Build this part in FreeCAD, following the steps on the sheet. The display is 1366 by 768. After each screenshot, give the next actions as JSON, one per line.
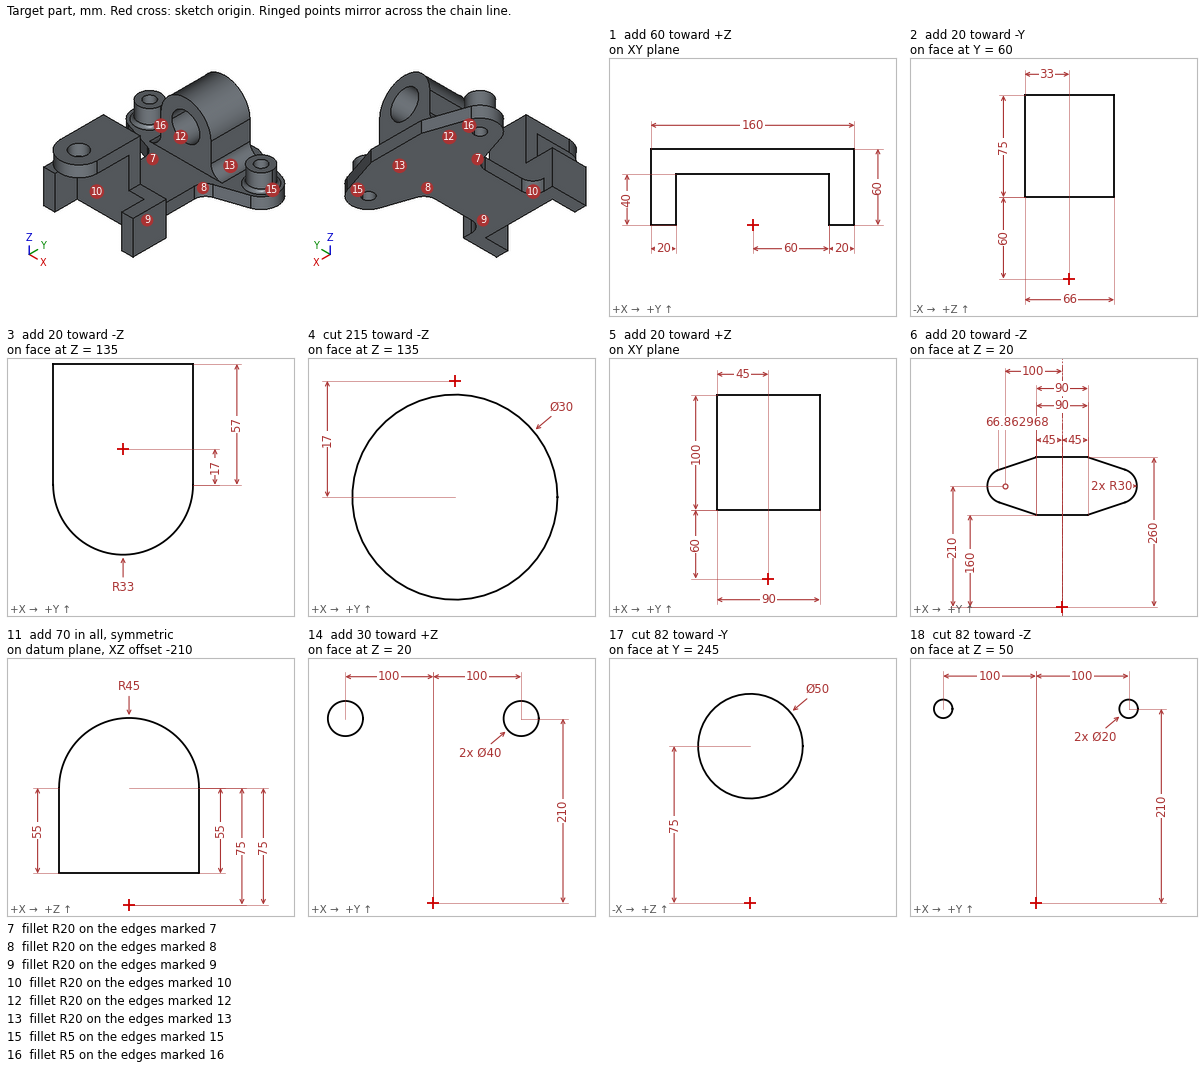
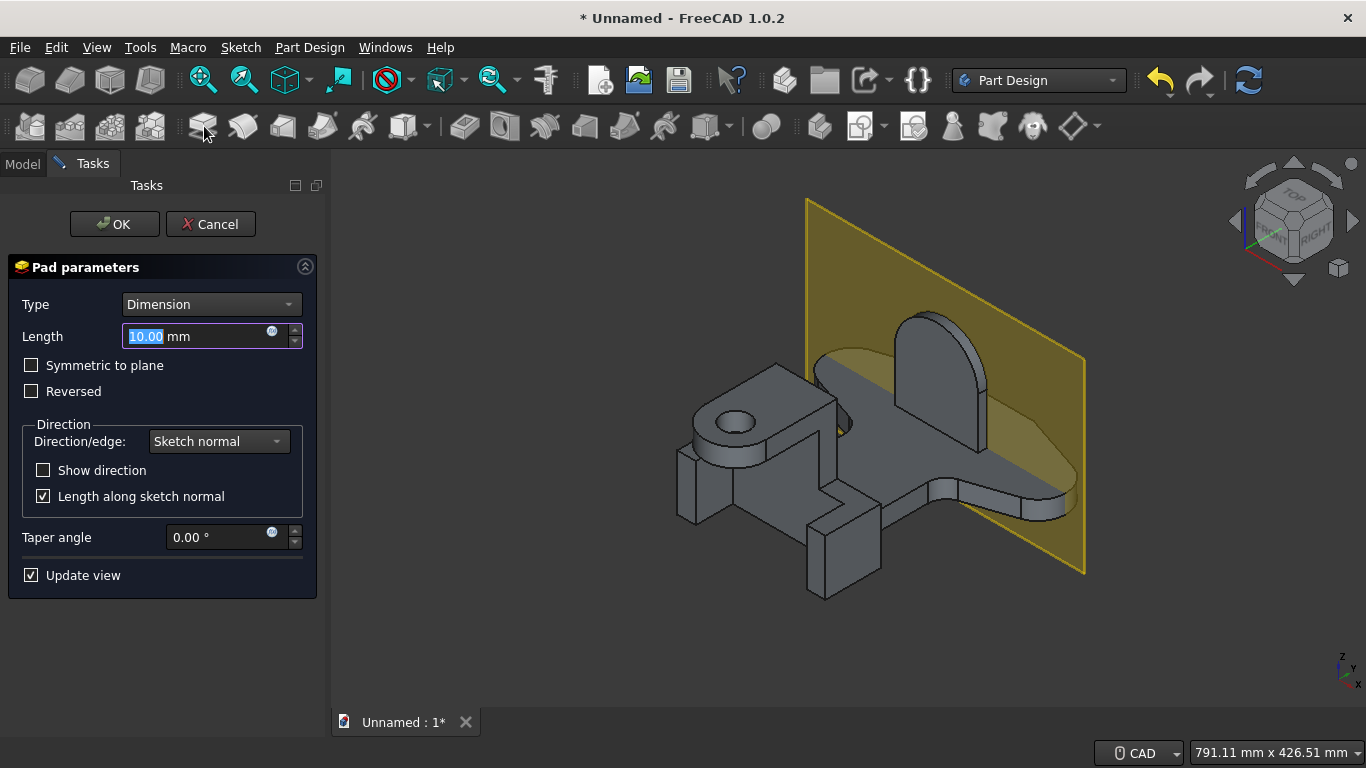
{"action": "type", "text": "70"}
{"action": "key", "text": "Tab"}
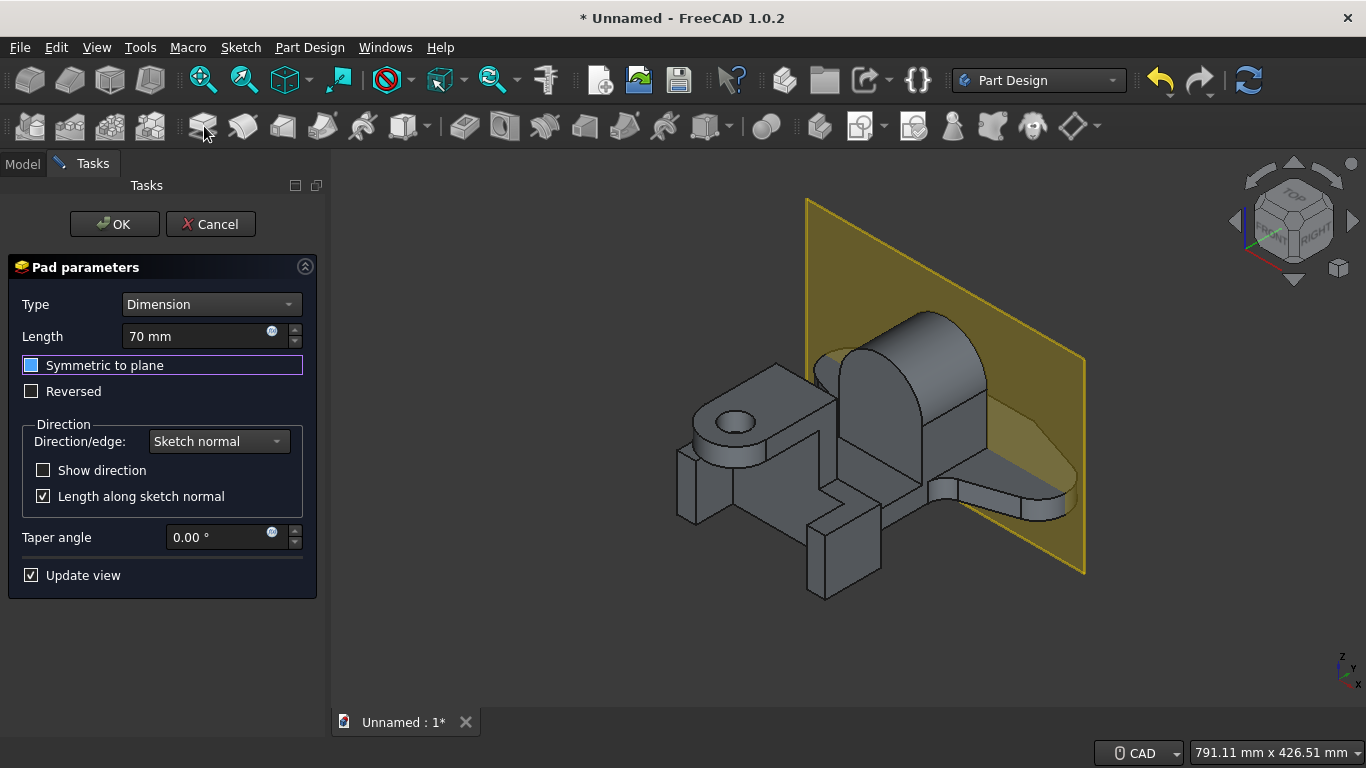
{"action": "left_click", "coordinate": [30, 365]}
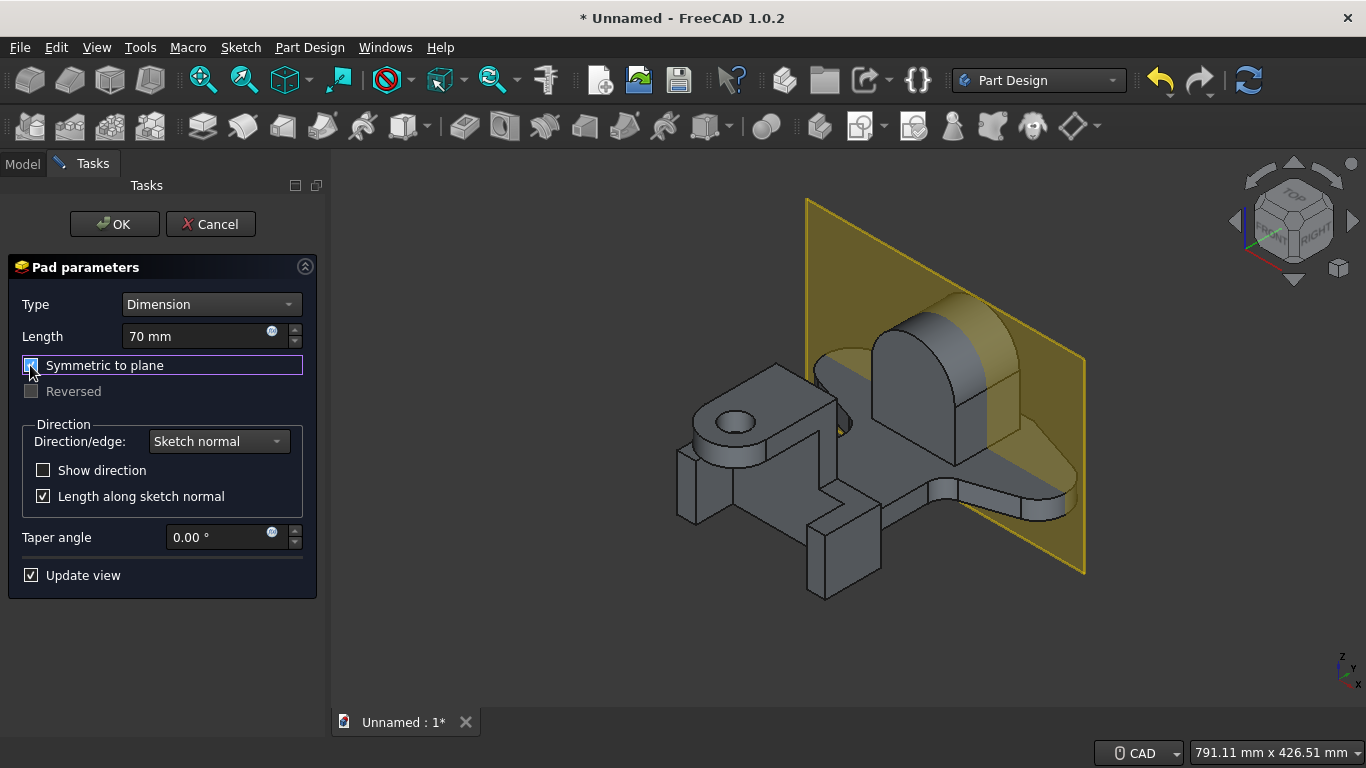
{"action": "left_click", "coordinate": [115, 224]}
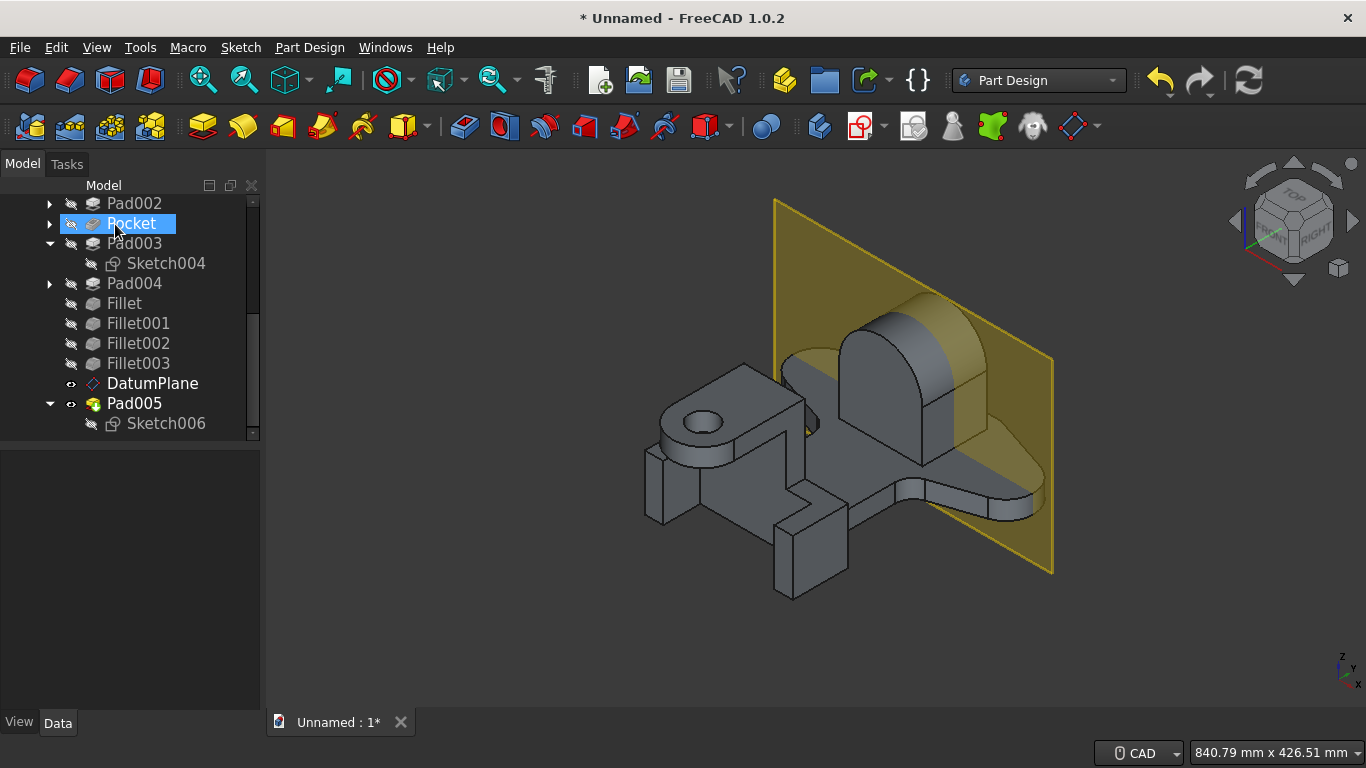
{"action": "left_click", "coordinate": [116, 384]}
{"action": "key", "text": "space"}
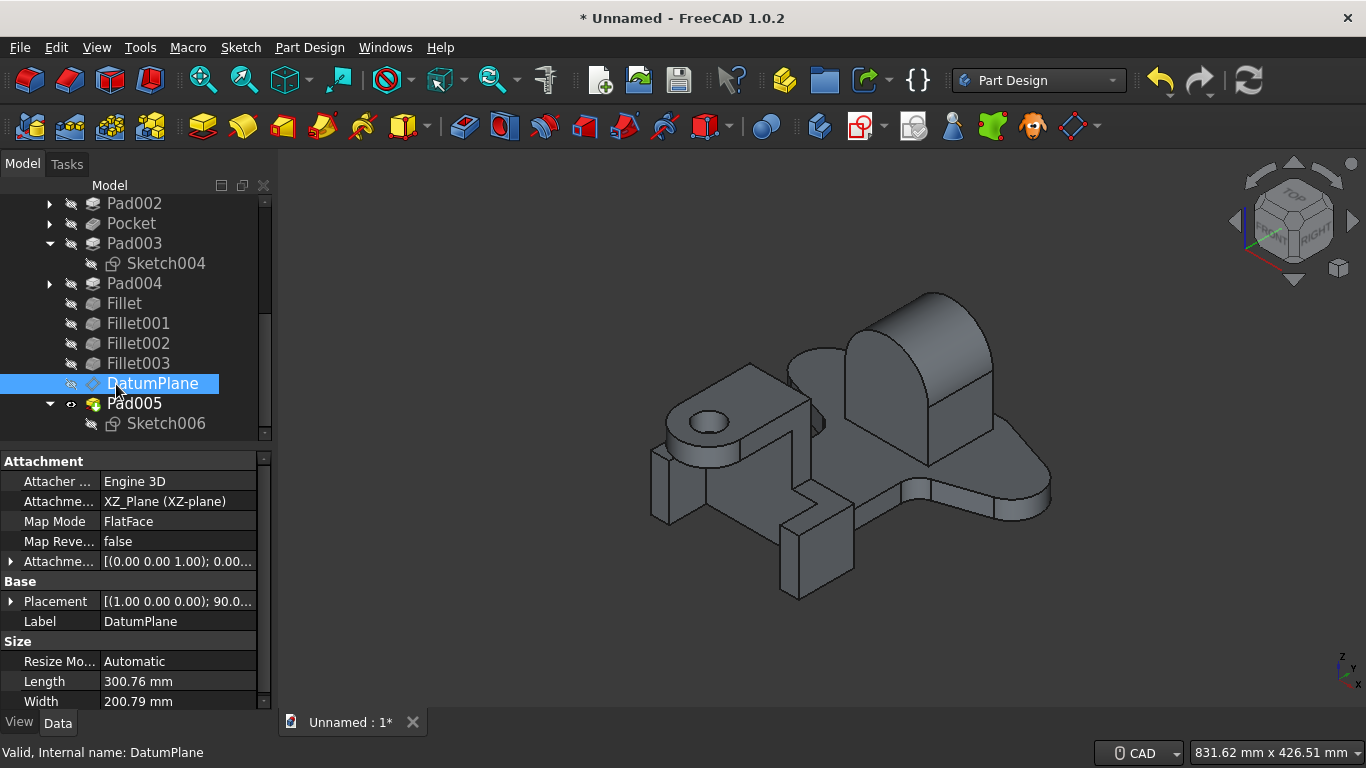
{"action": "key", "text": "2"}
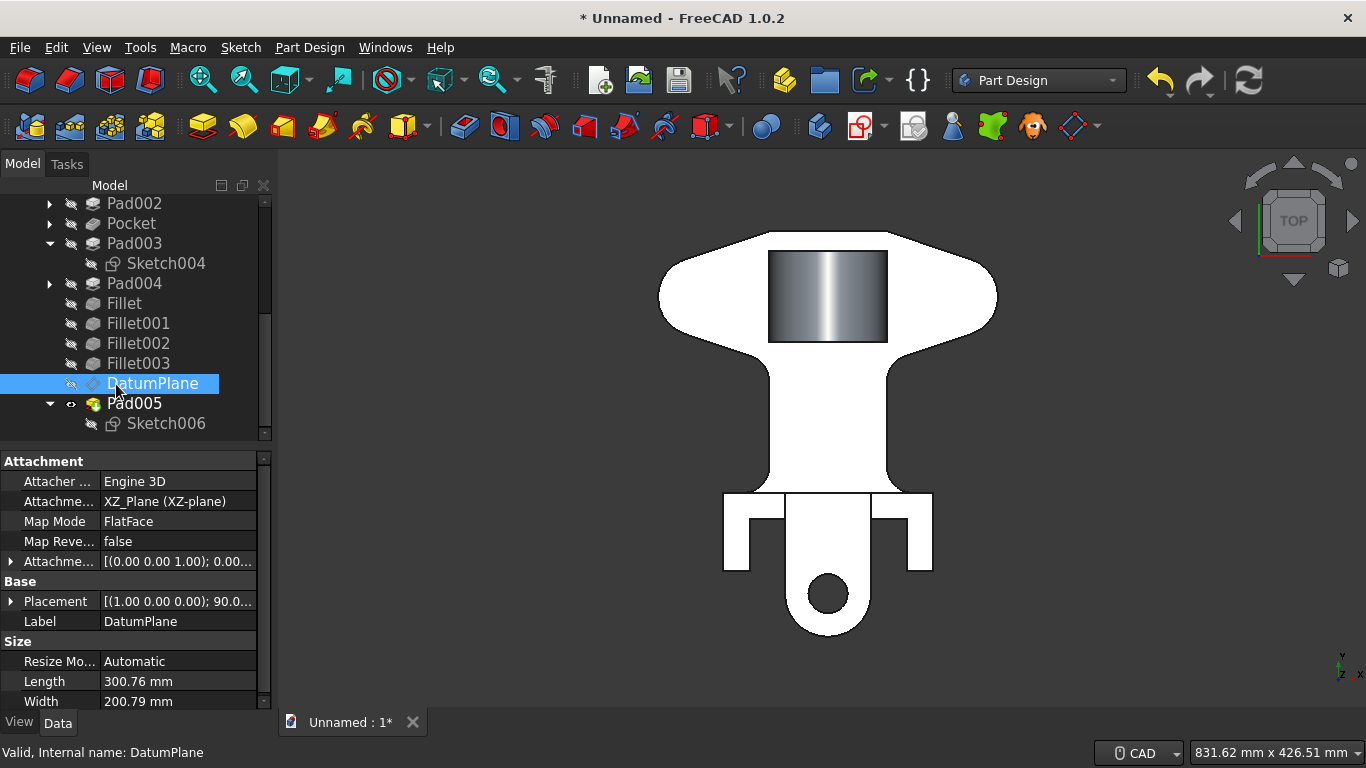
{"action": "key", "text": "0"}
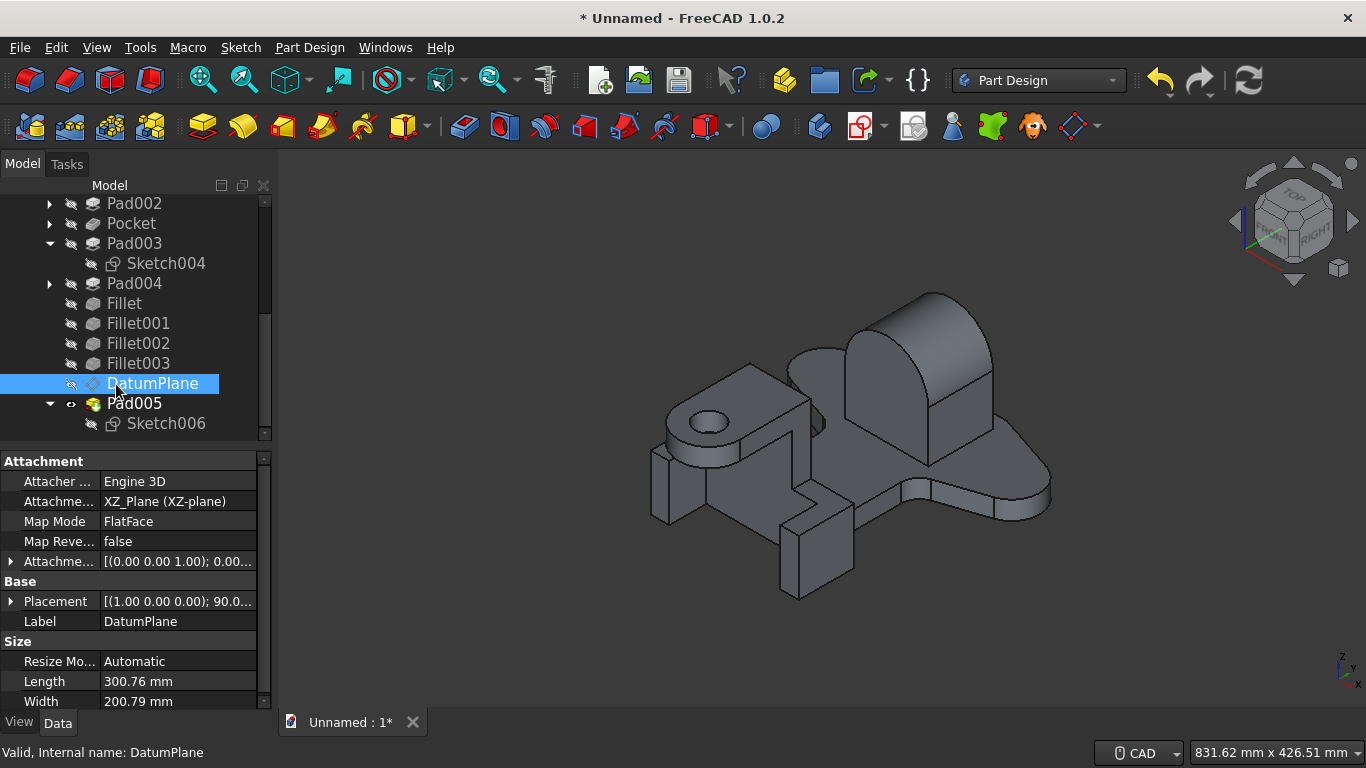
{"action": "key", "text": "1"}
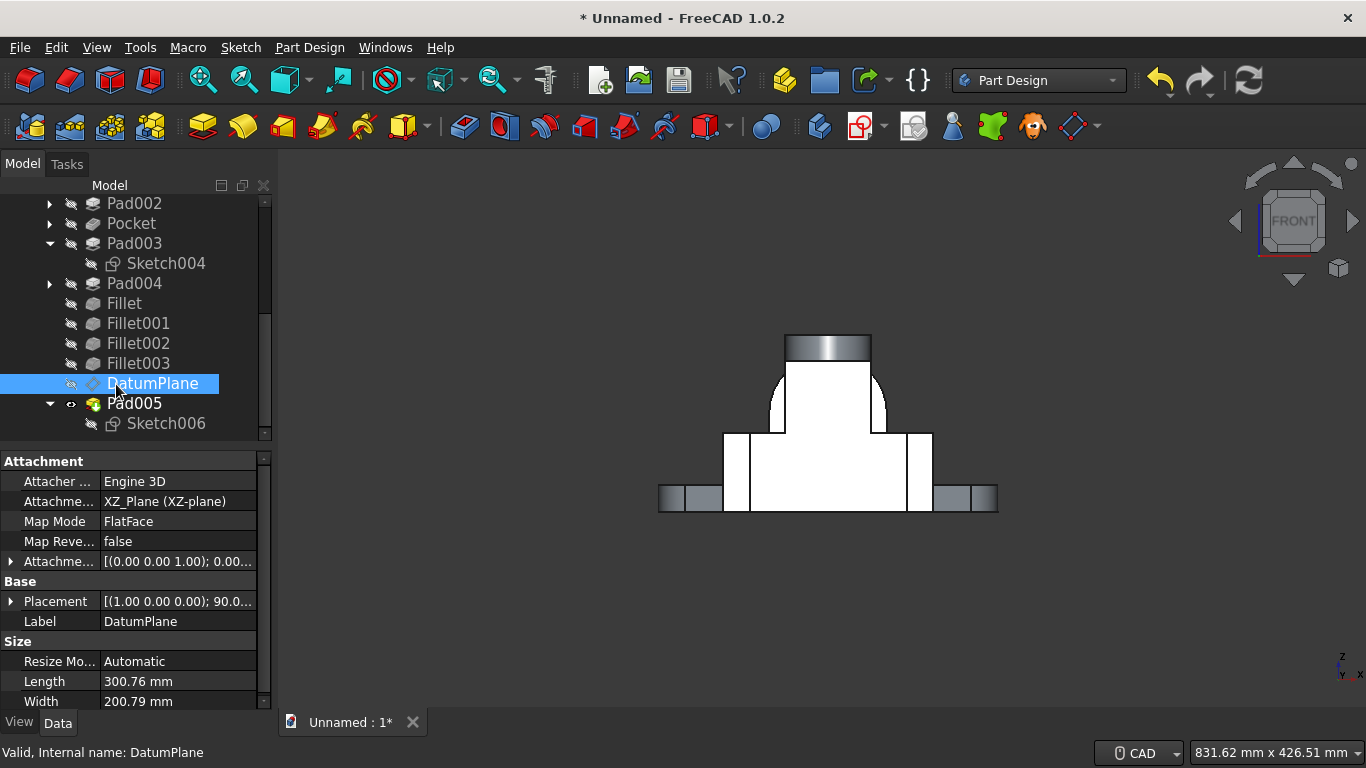
{"action": "key", "text": "v f"}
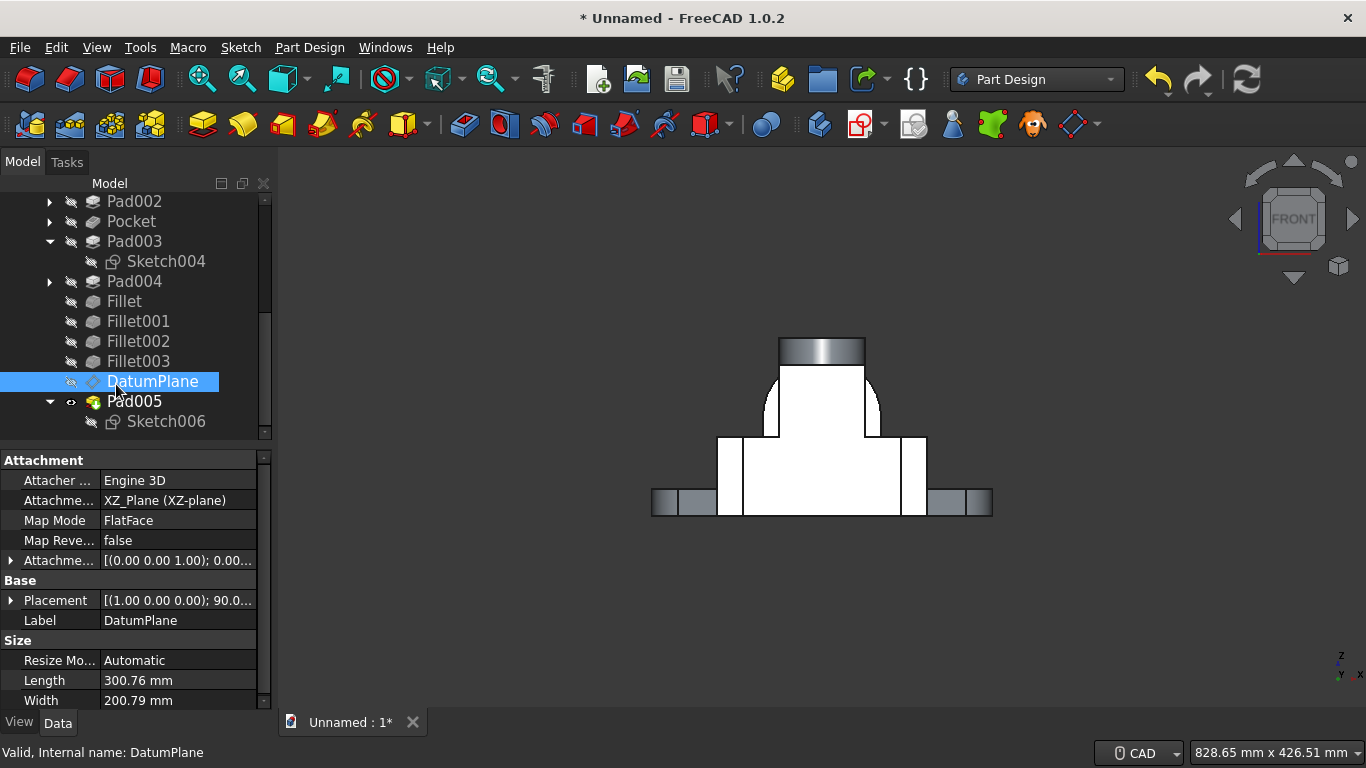
{"action": "key", "text": "3"}